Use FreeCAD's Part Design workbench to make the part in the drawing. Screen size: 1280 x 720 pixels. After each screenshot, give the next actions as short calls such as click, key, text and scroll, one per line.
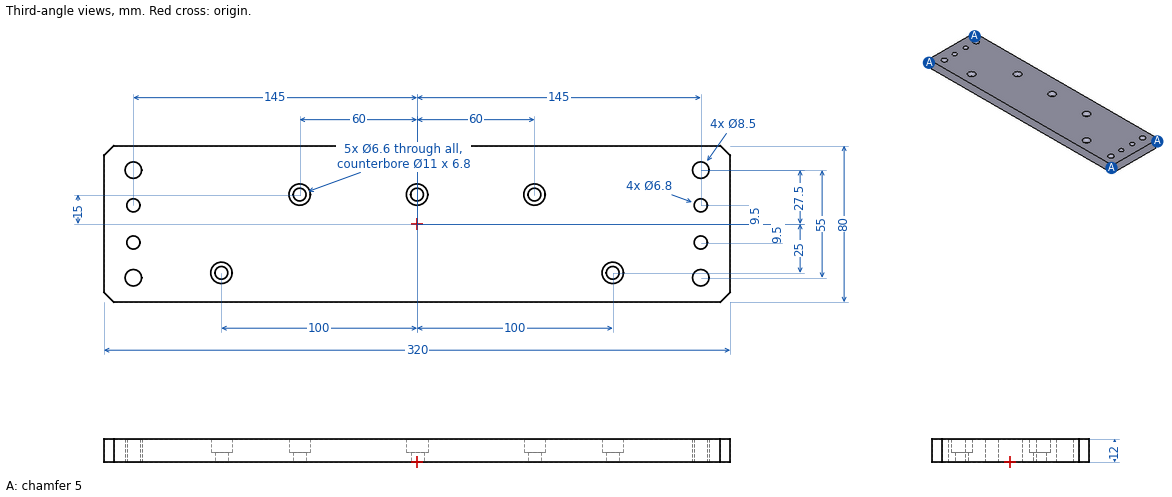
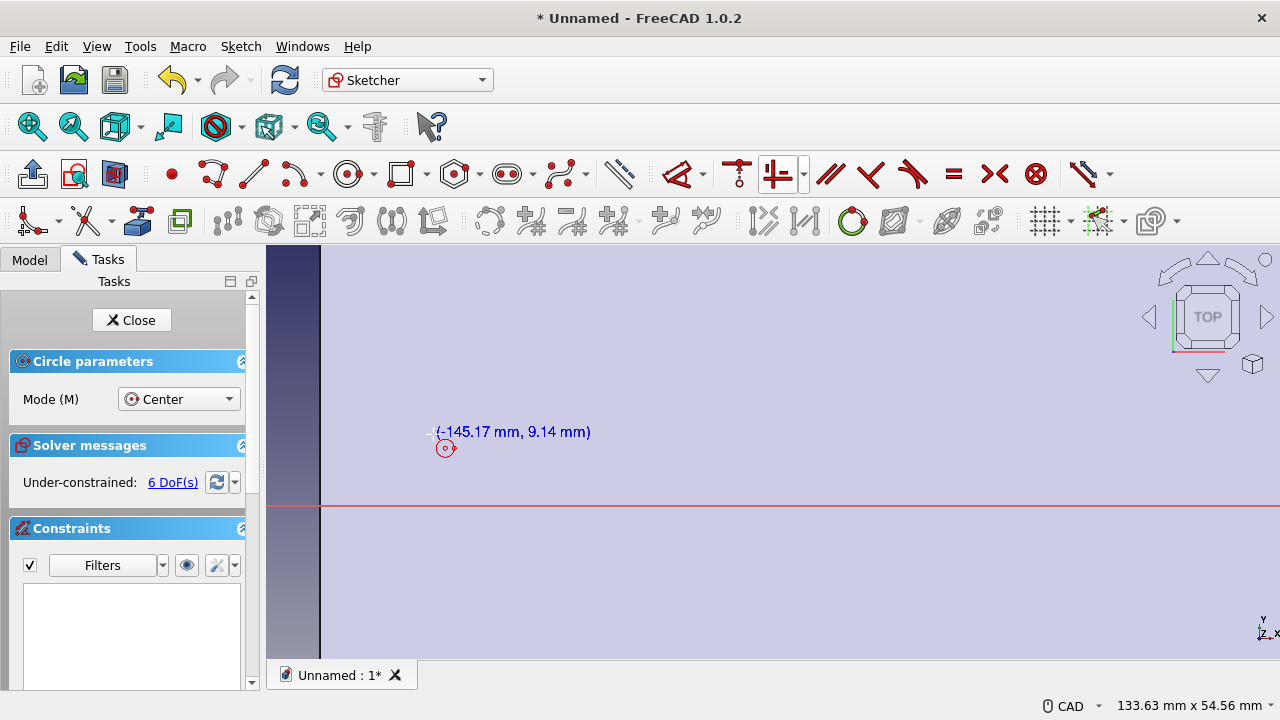
scroll(433, 434, down, 7)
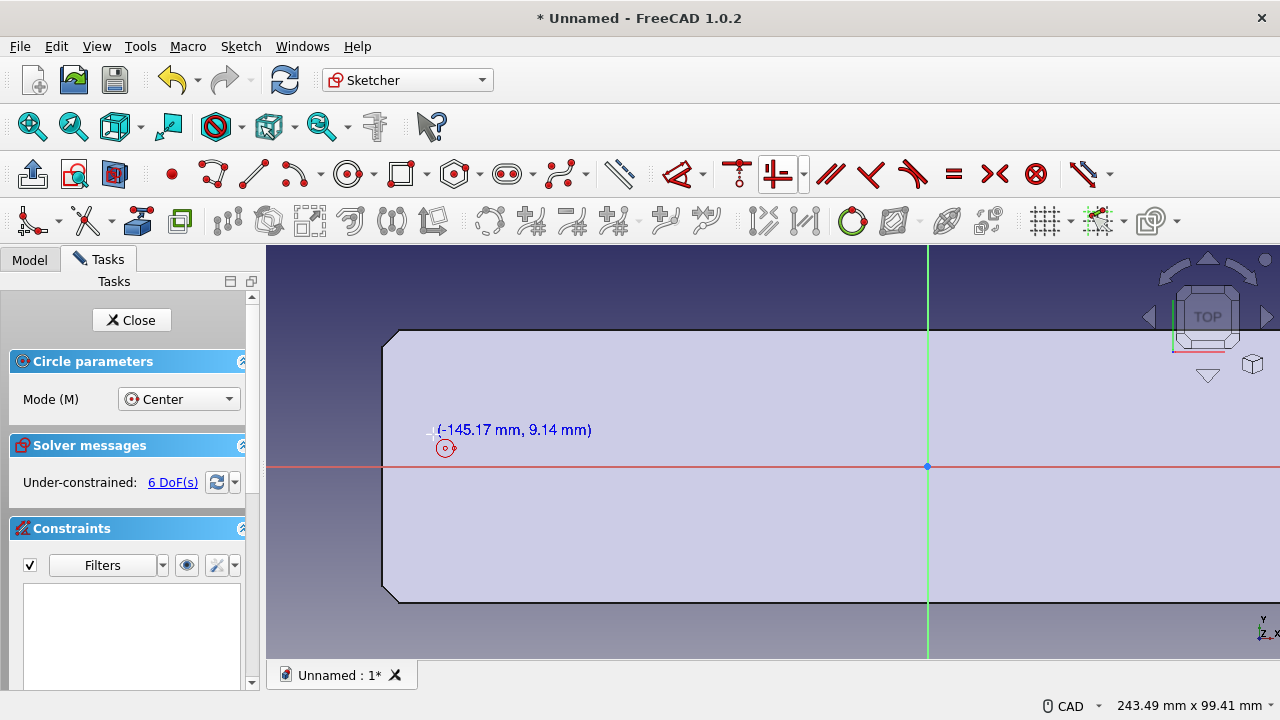
click(433, 434)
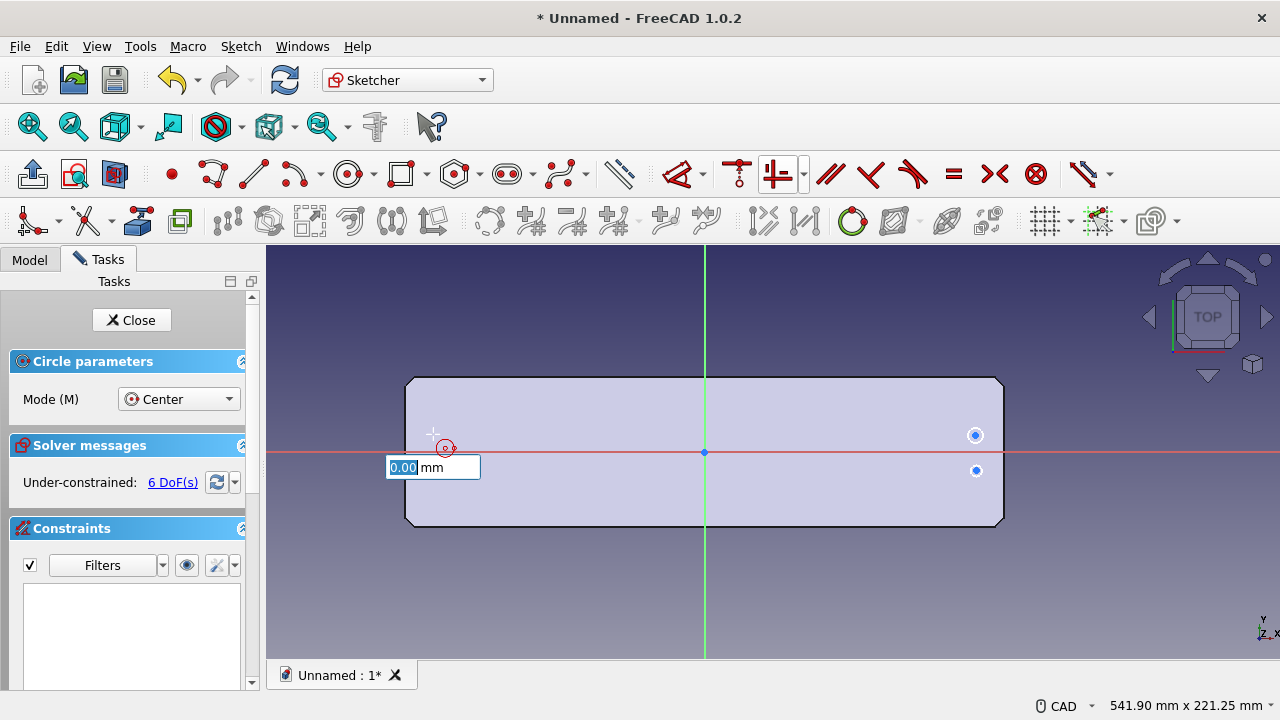
scroll(438, 430, up, 5)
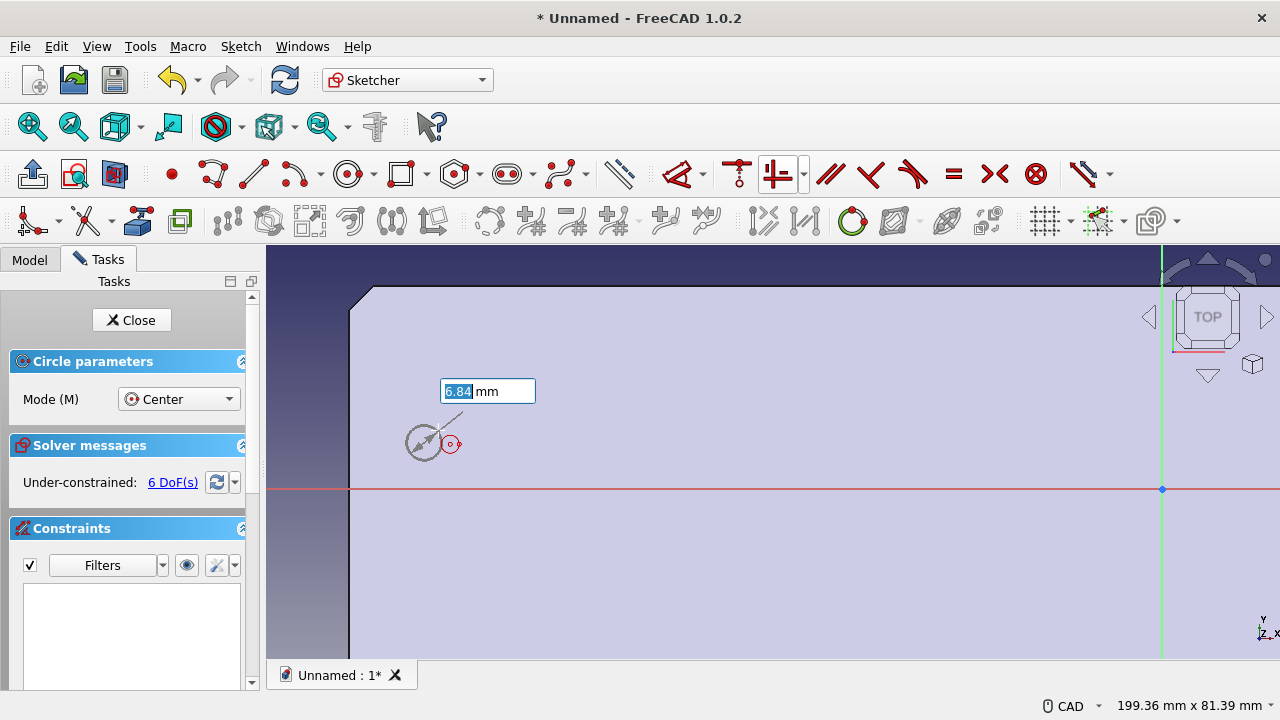
click(437, 429)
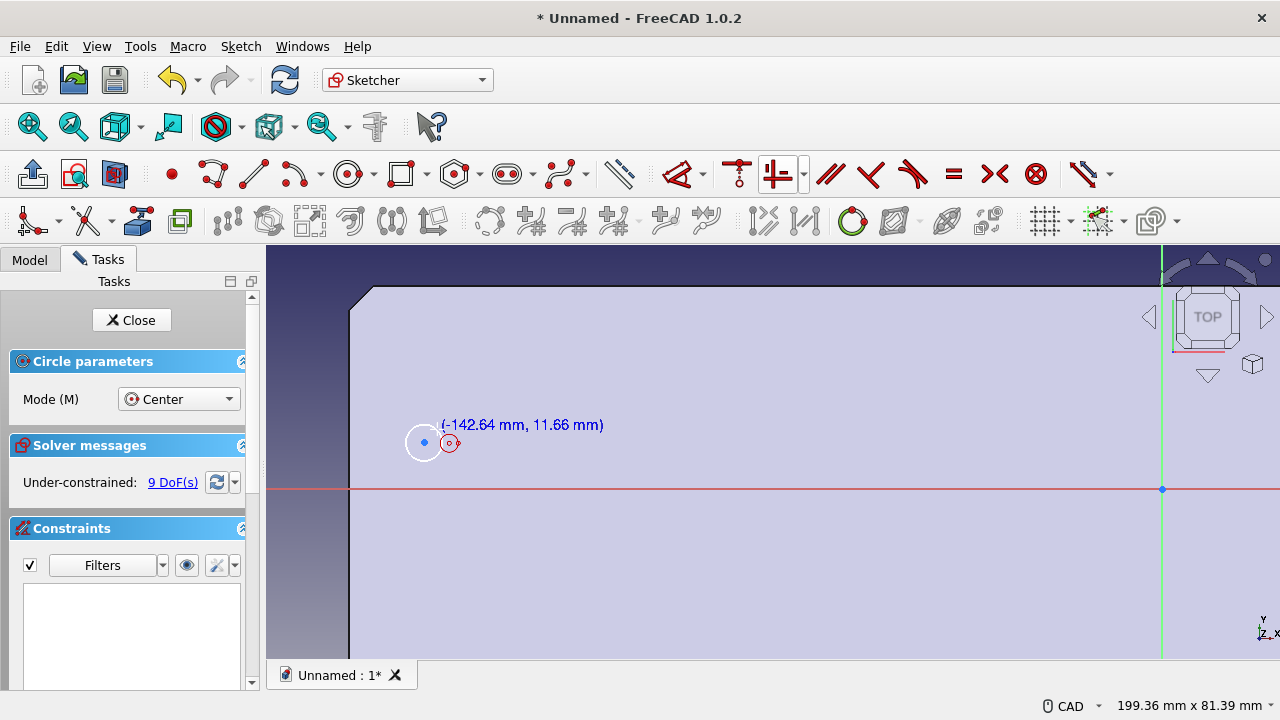
scroll(425, 538, up, 2)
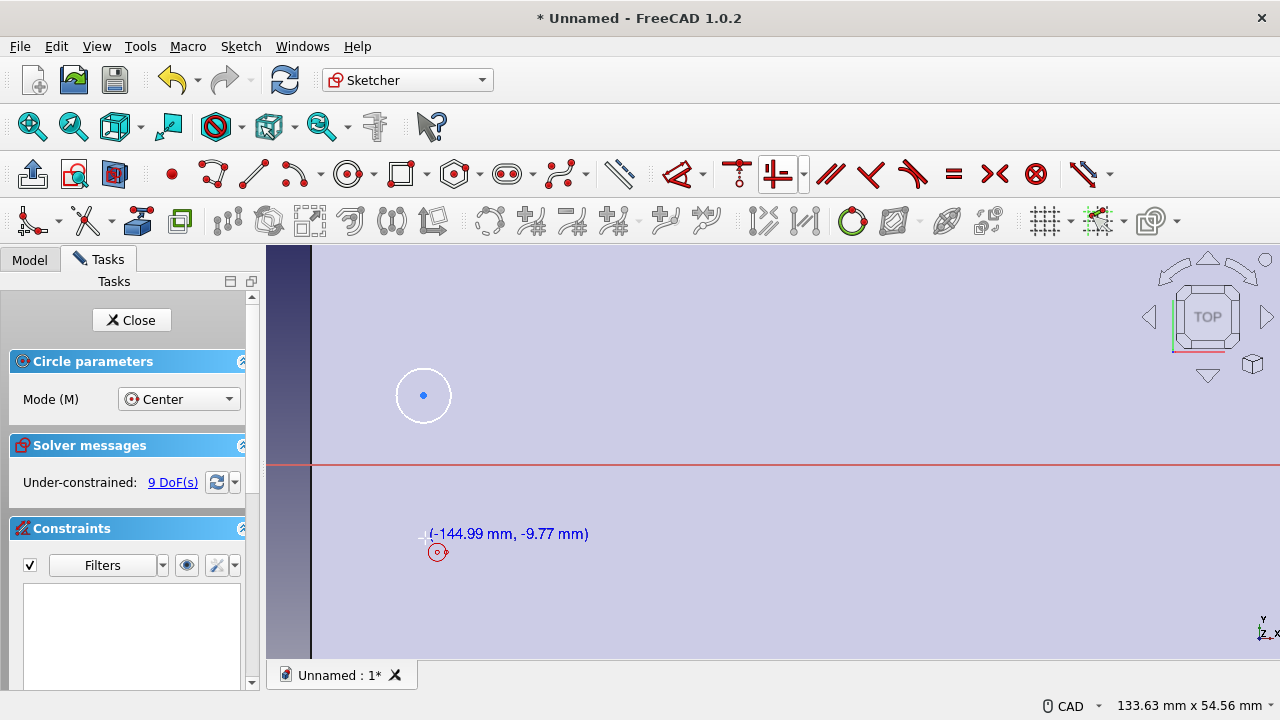
scroll(436, 448, down, 7)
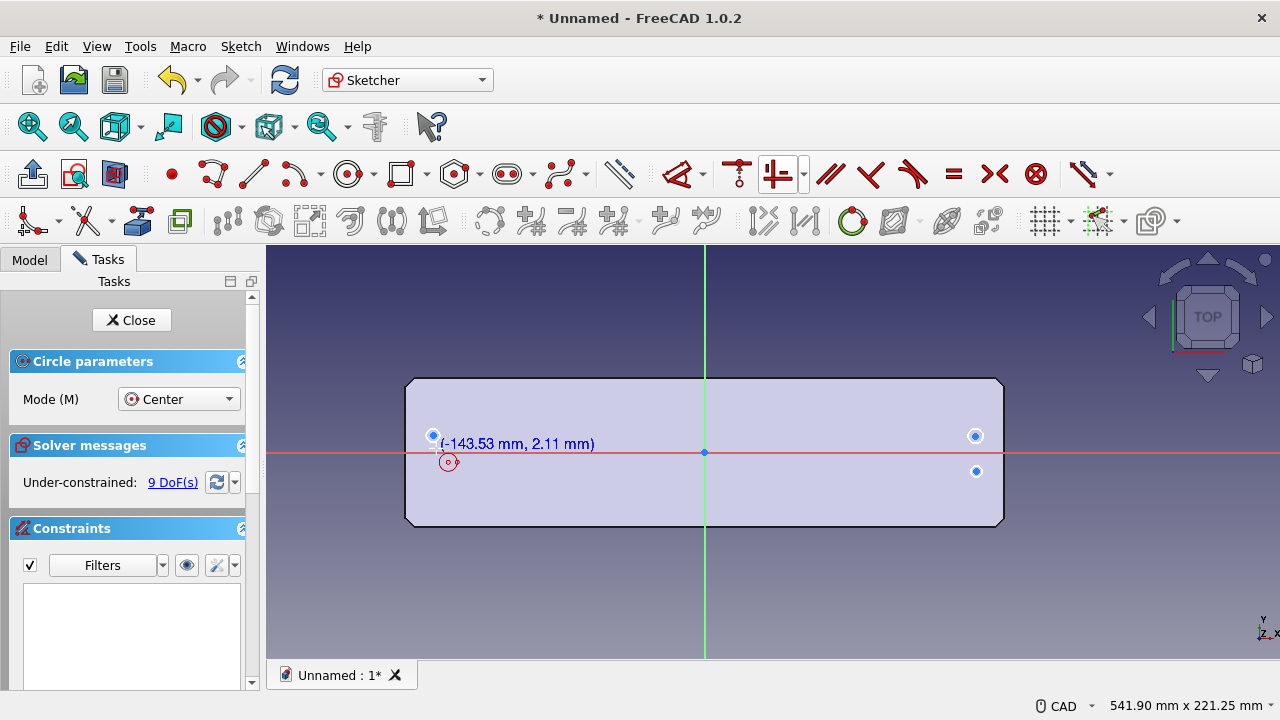
click(433, 470)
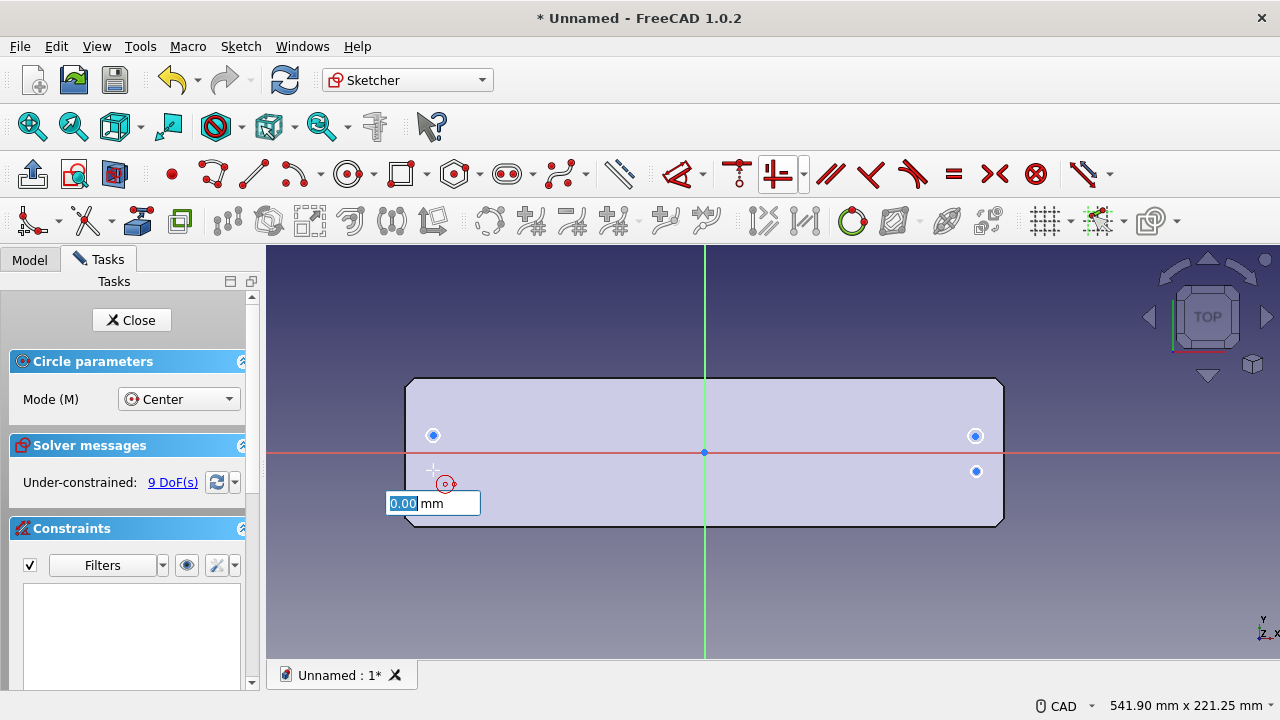
scroll(438, 475, up, 5)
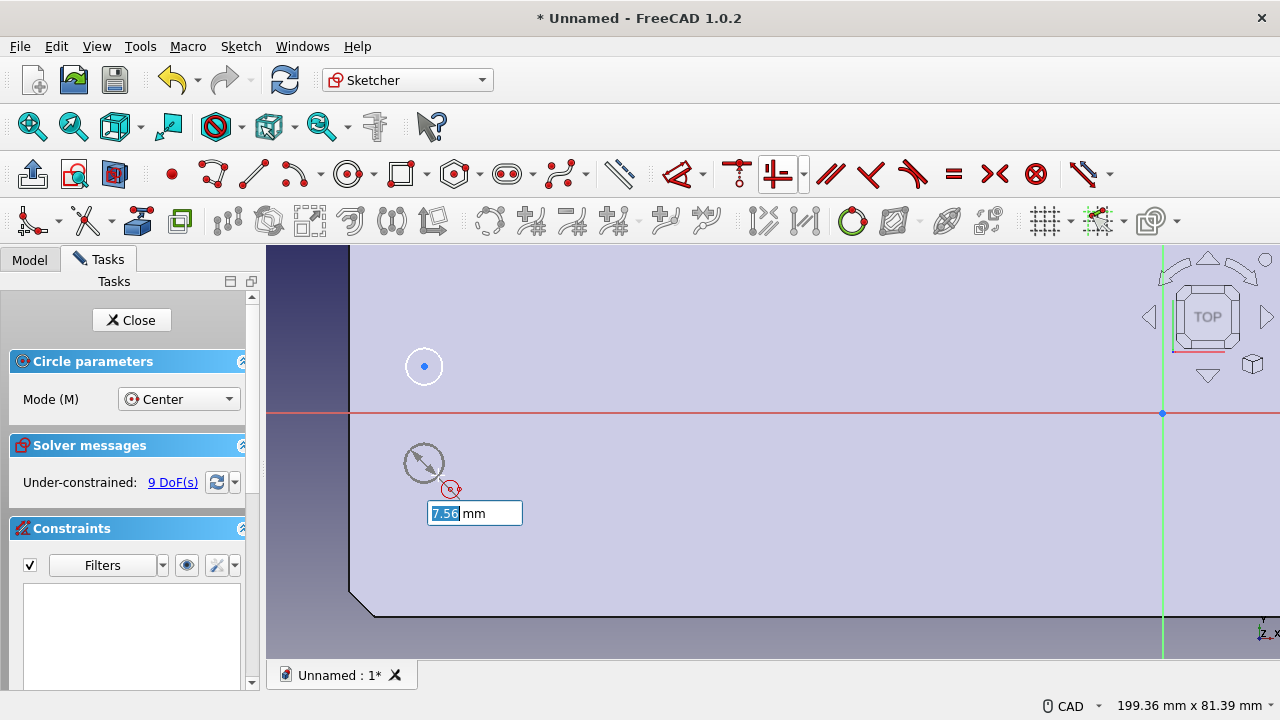
click(437, 474)
key(Escape)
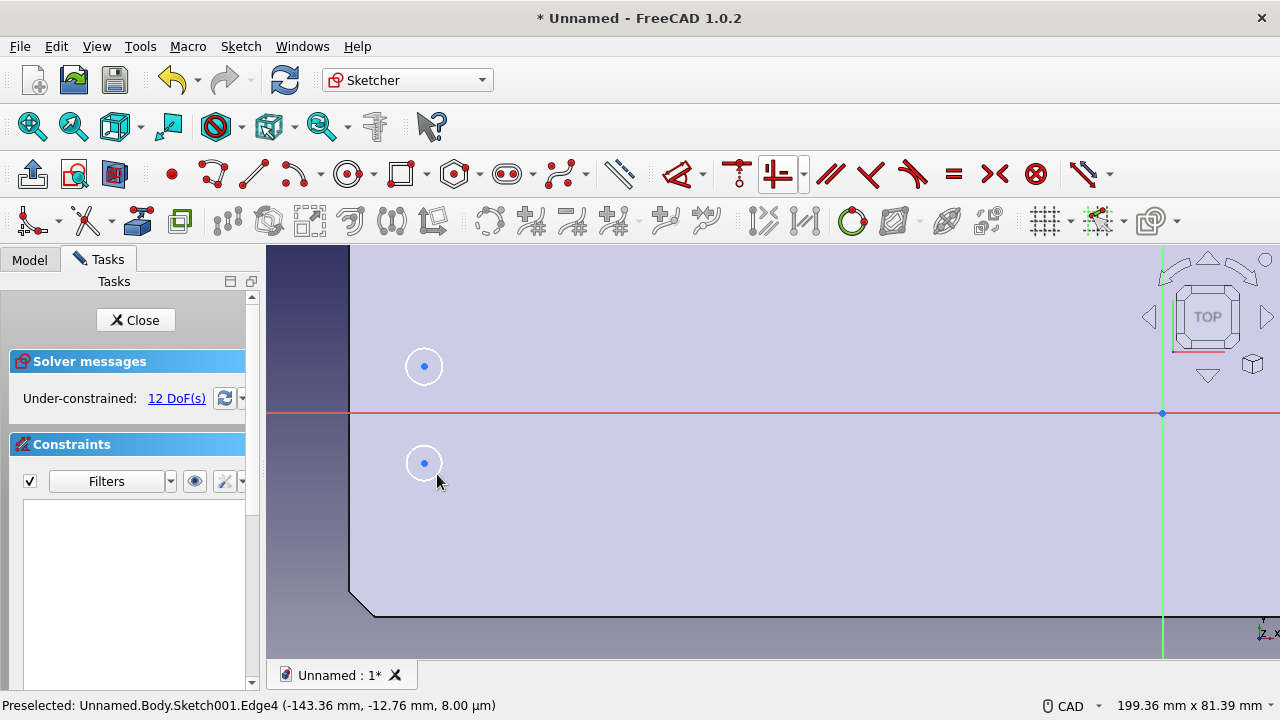
scroll(438, 475, down, 5)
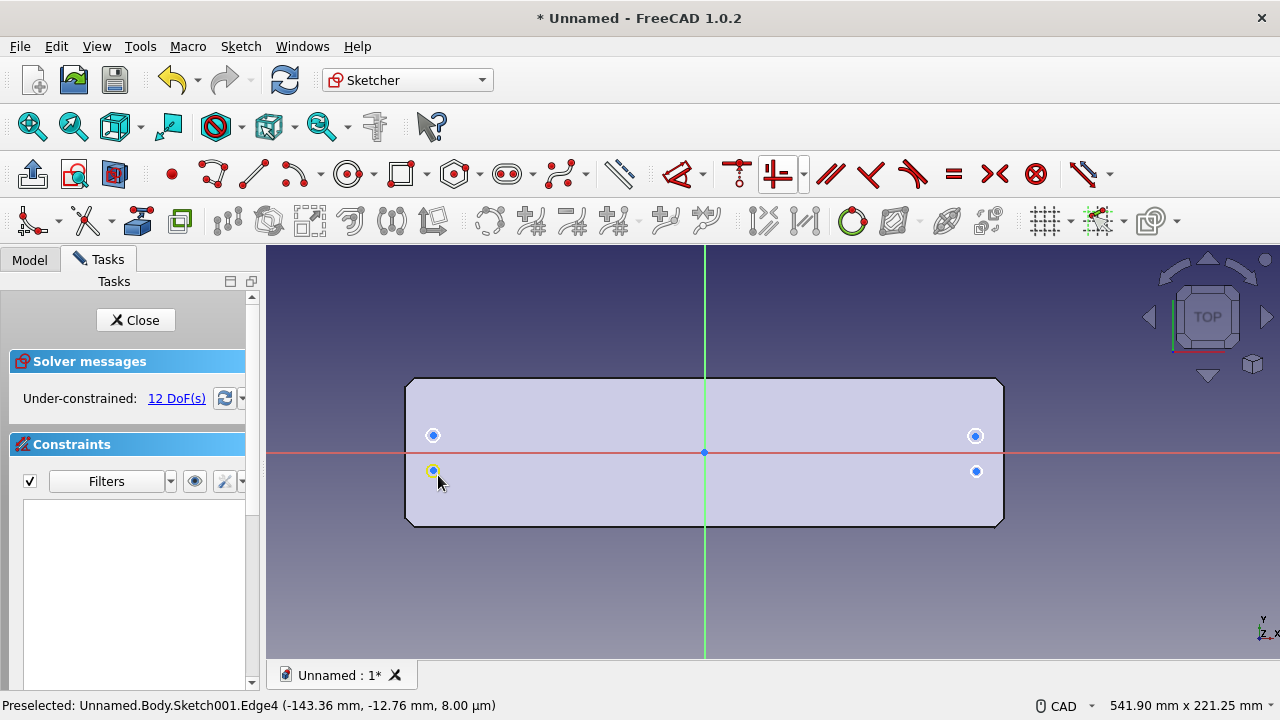
scroll(981, 431, up, 4)